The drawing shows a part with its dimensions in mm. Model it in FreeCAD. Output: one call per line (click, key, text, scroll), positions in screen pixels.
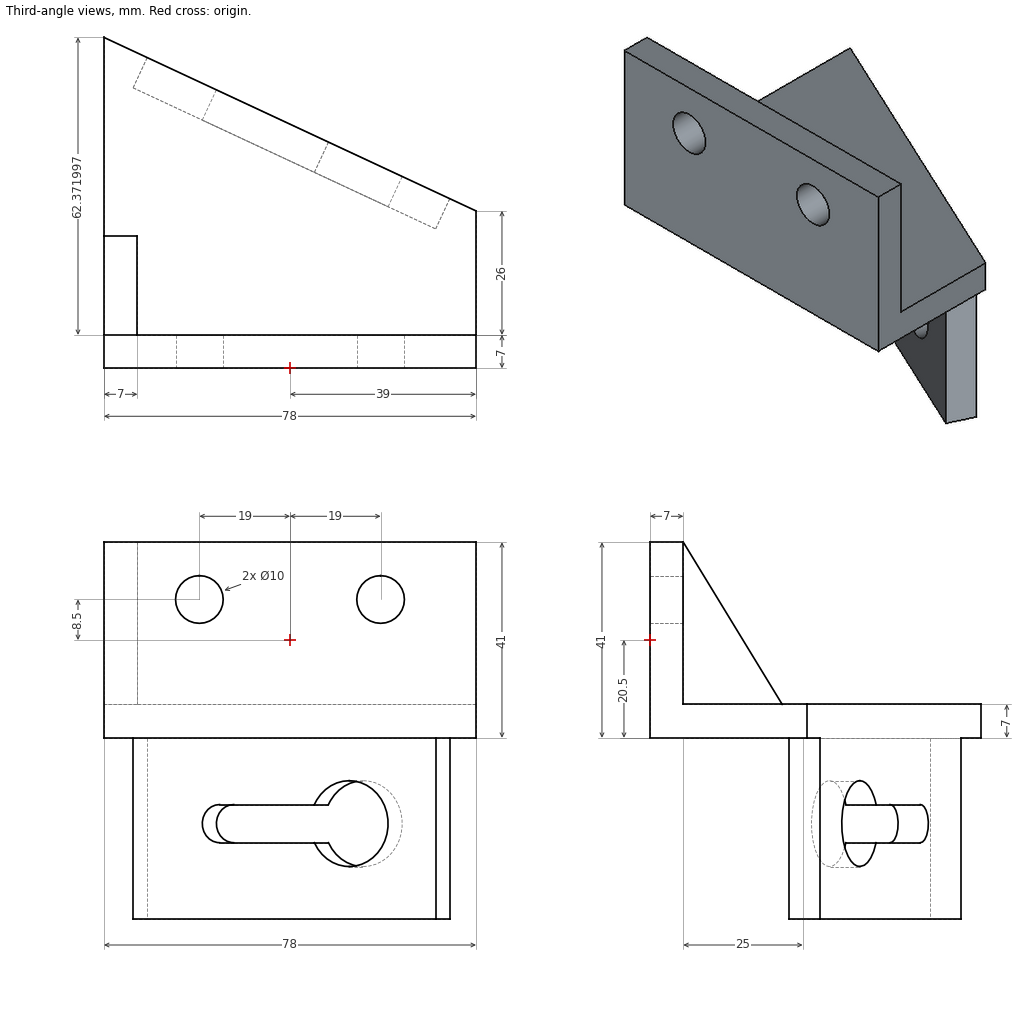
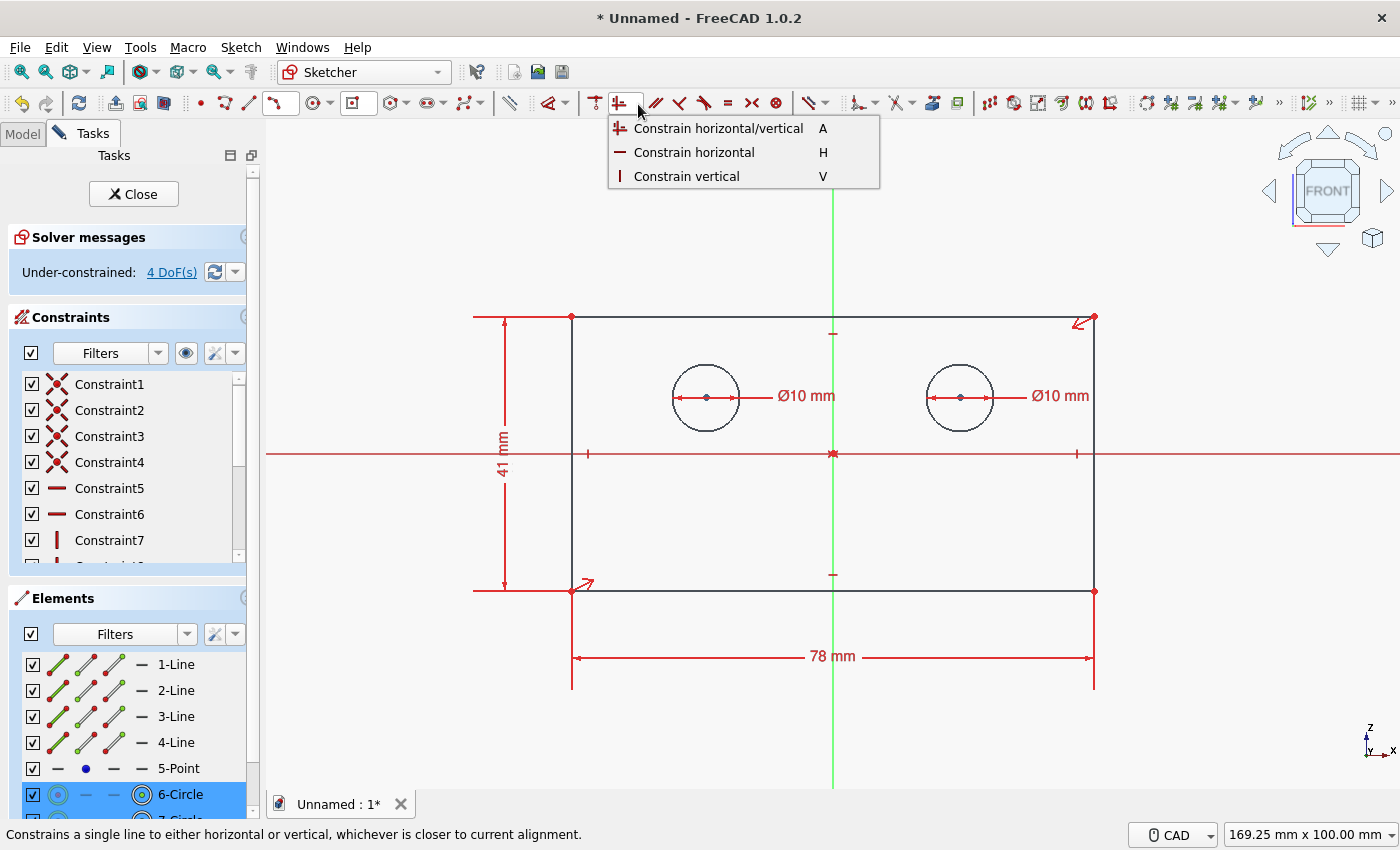
click(744, 152)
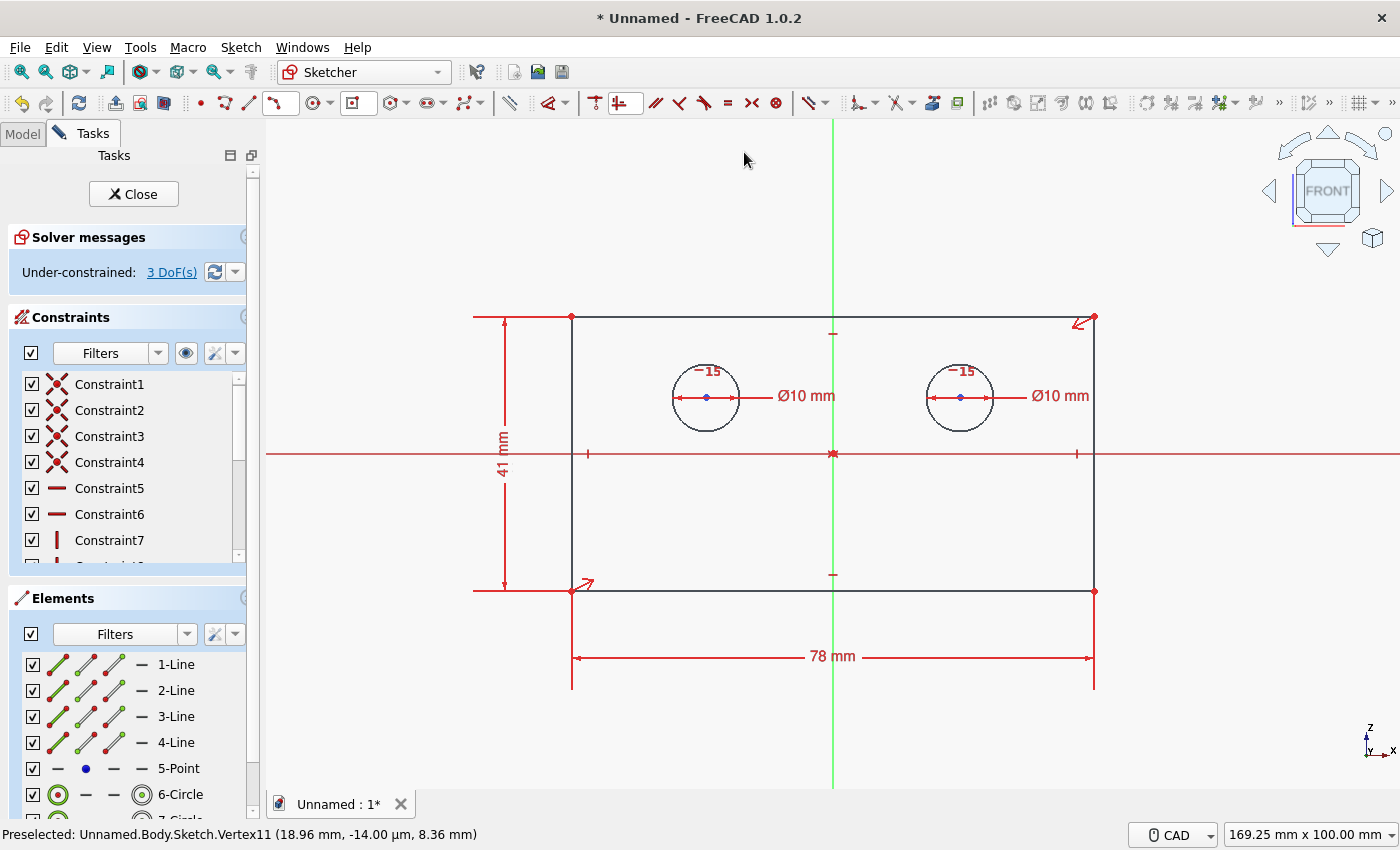
click(548, 104)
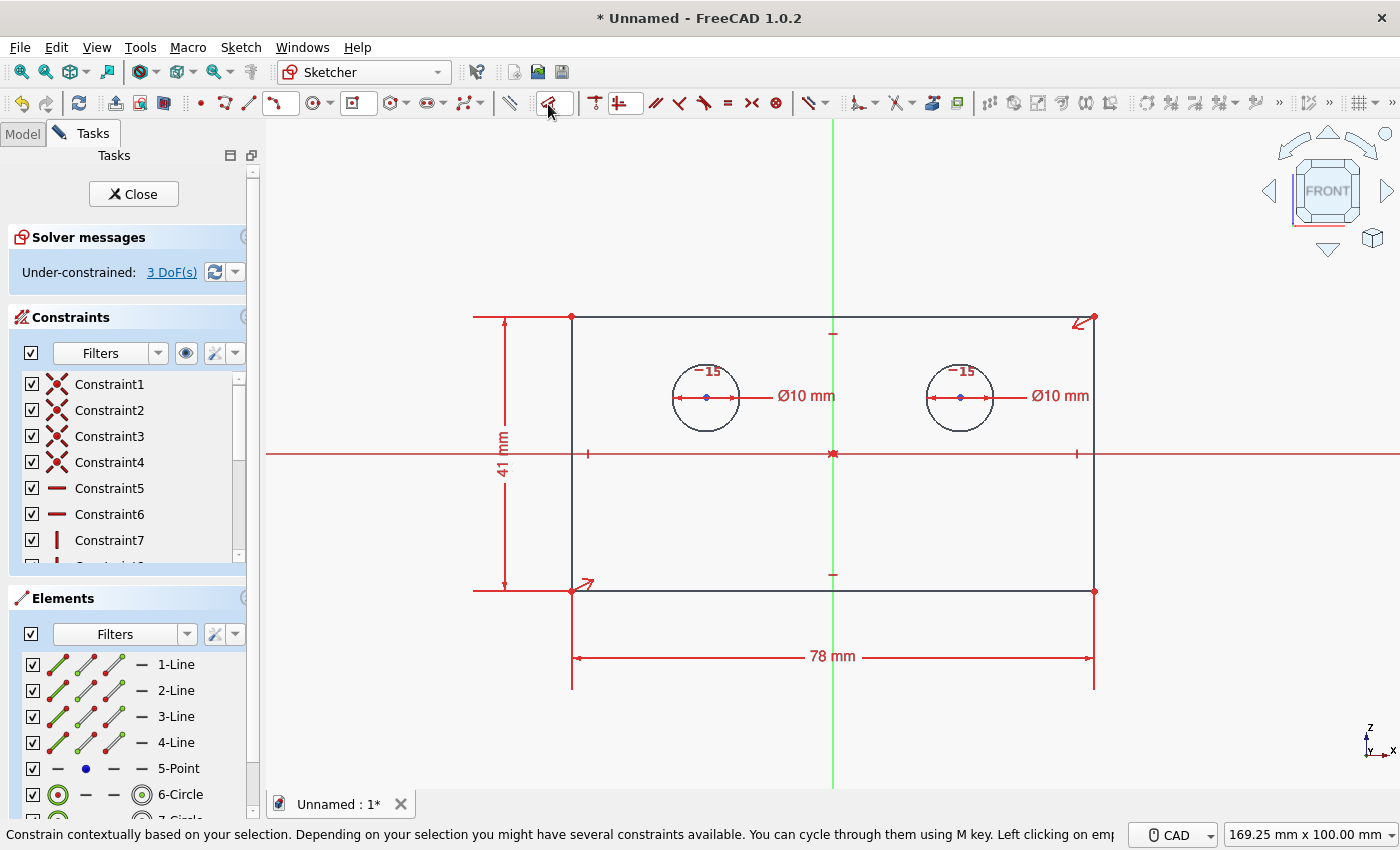
click(706, 398)
click(769, 364)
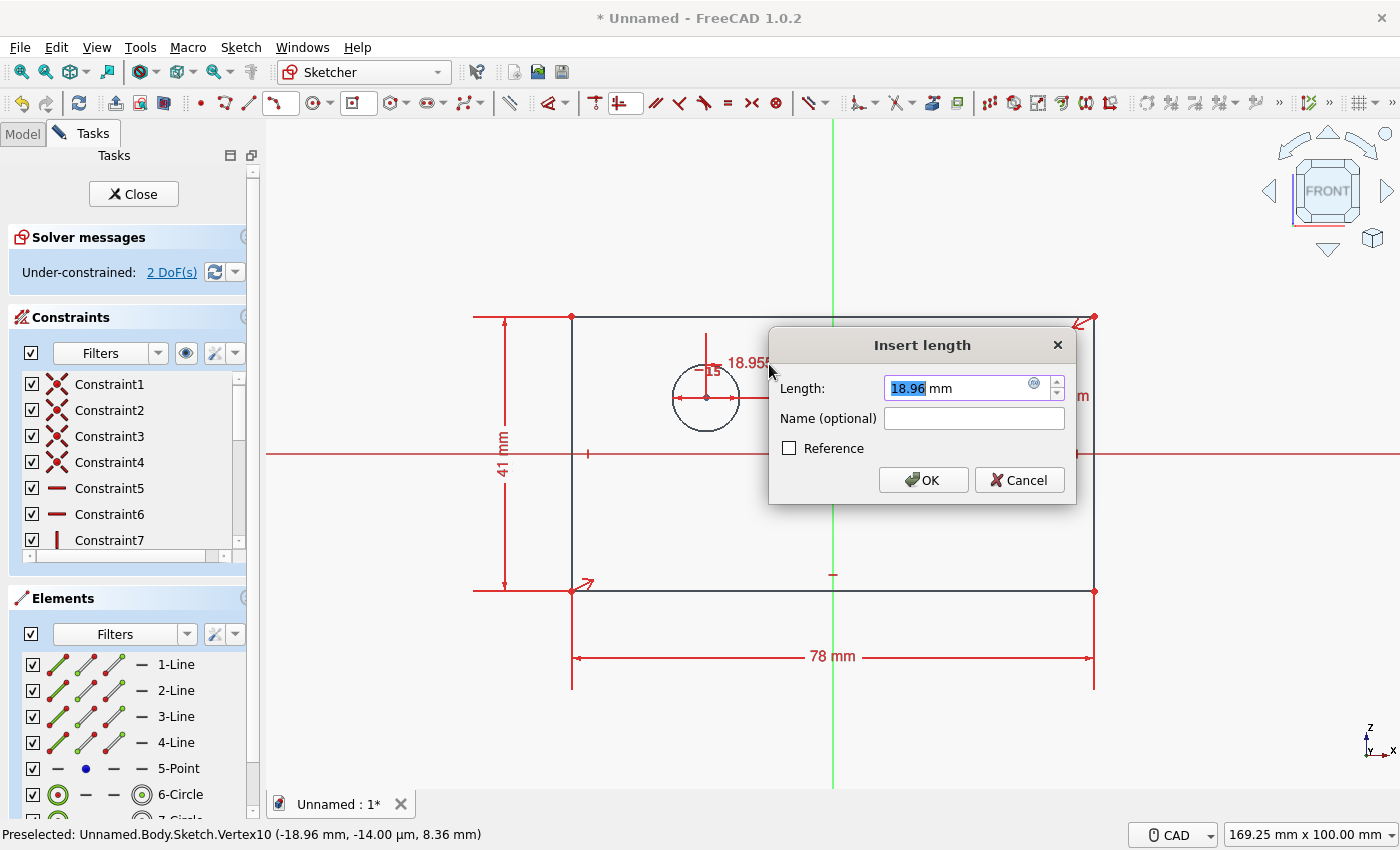
text(19)
key(Return)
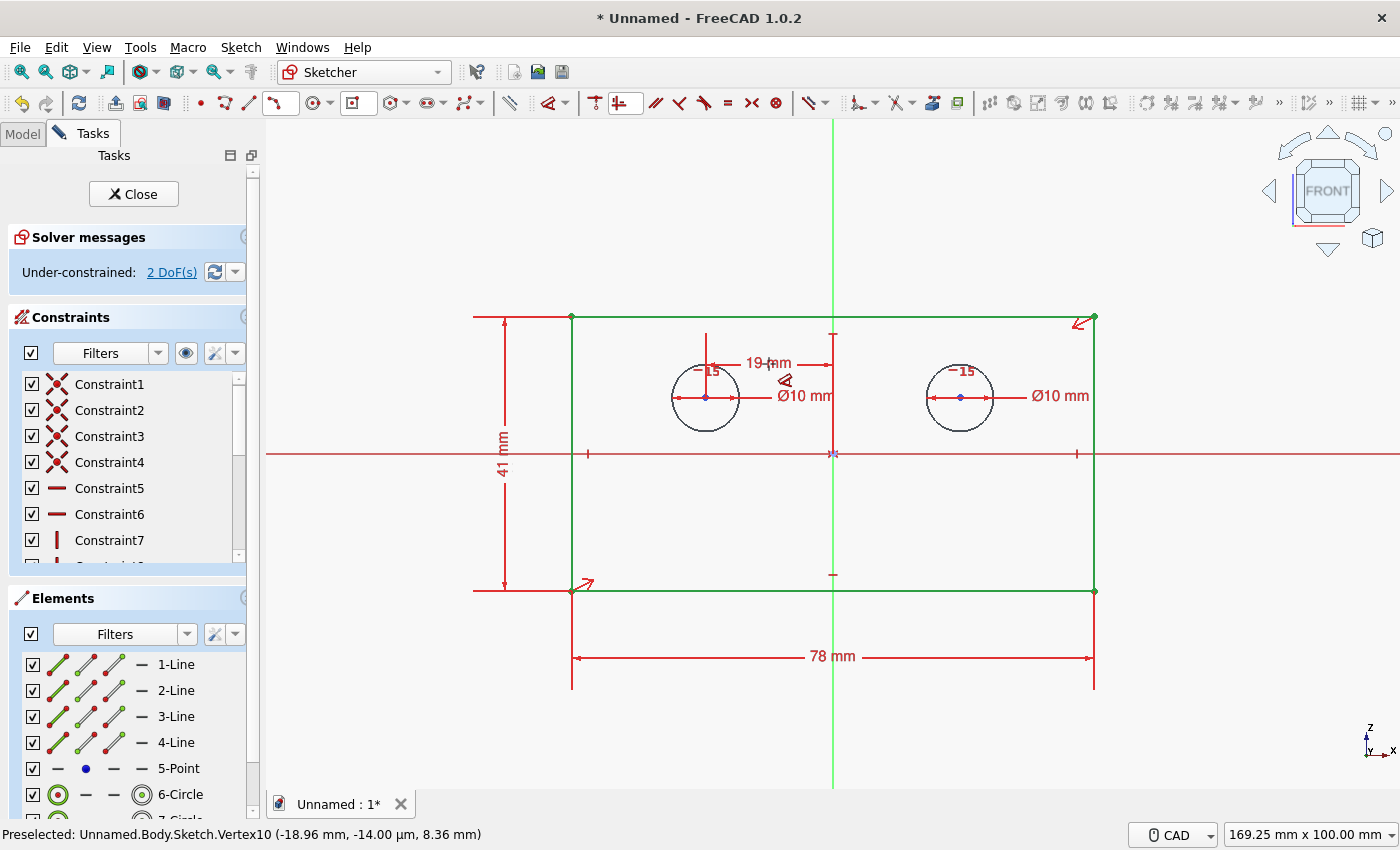
click(960, 398)
click(897, 364)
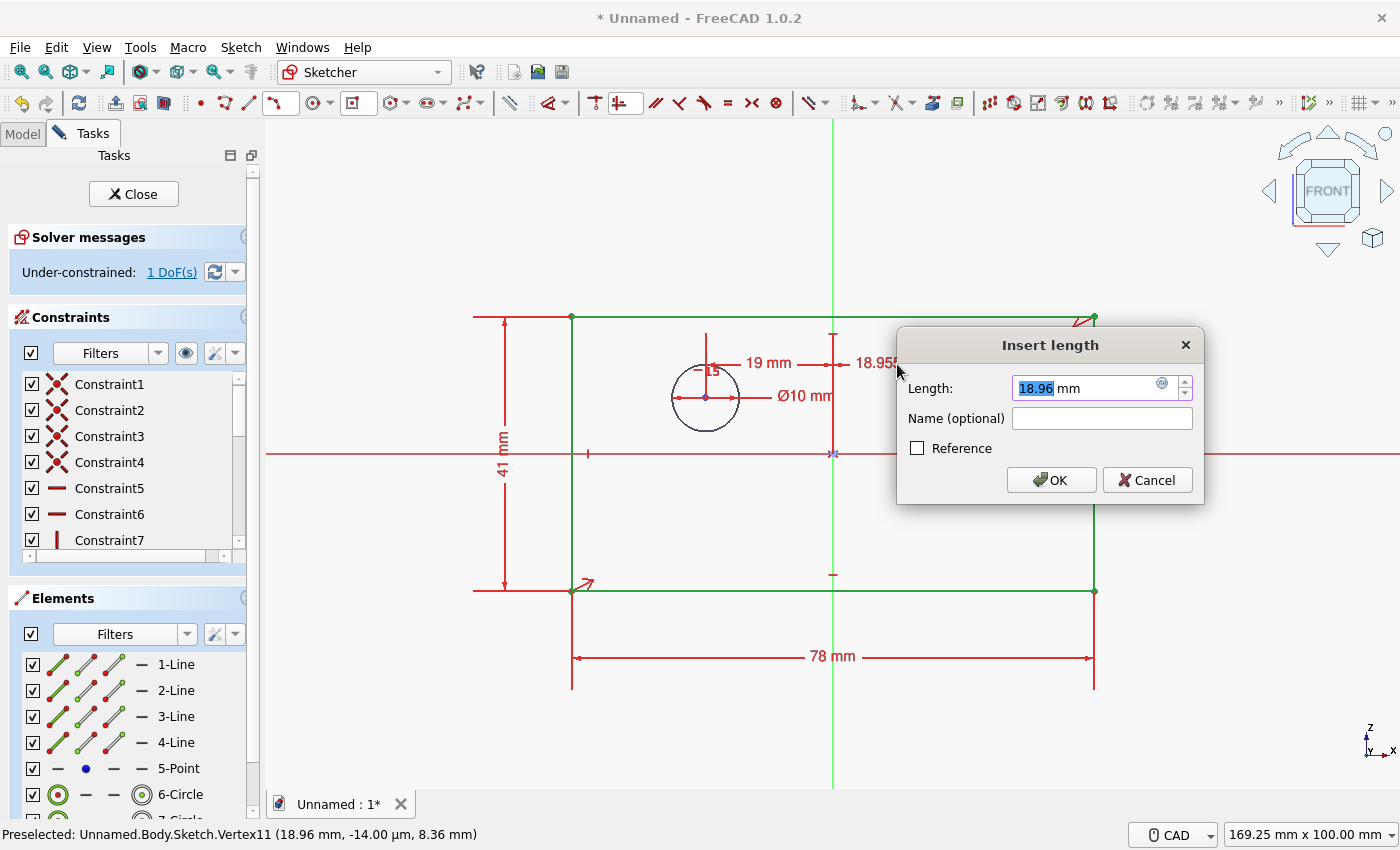
text(19)
key(Return)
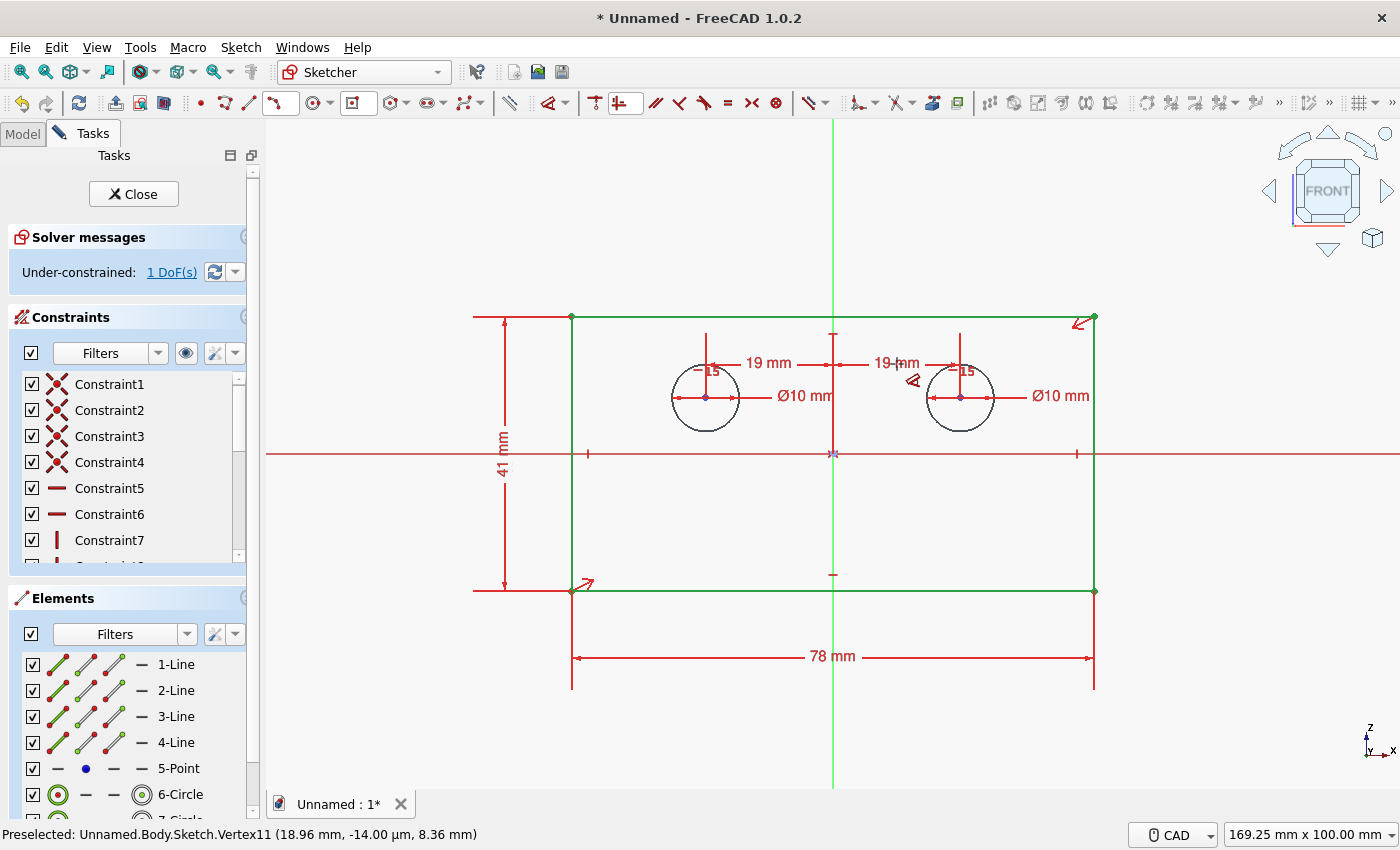
click(706, 398)
click(672, 439)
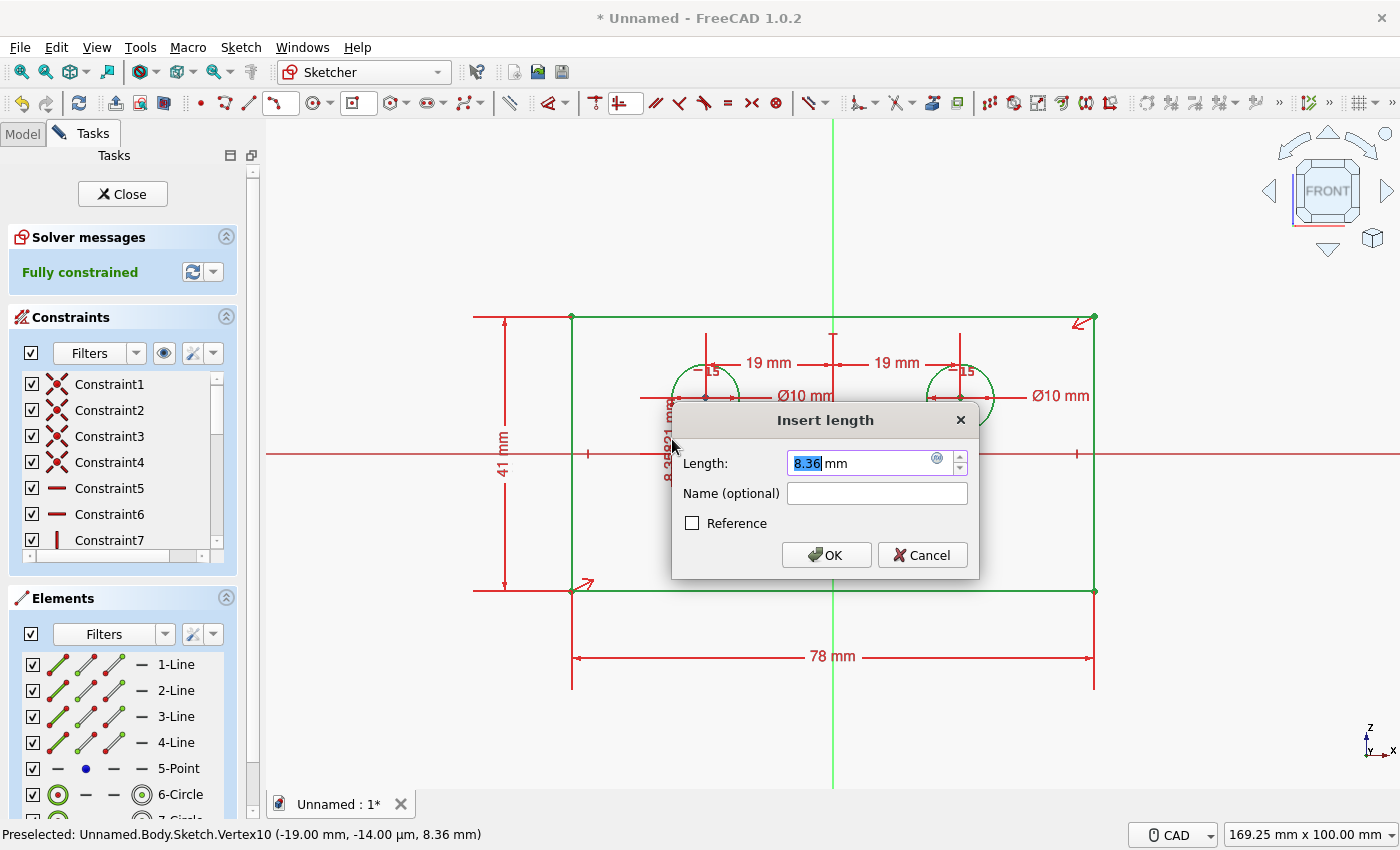
text(8.5)
key(Return)
key(Escape)